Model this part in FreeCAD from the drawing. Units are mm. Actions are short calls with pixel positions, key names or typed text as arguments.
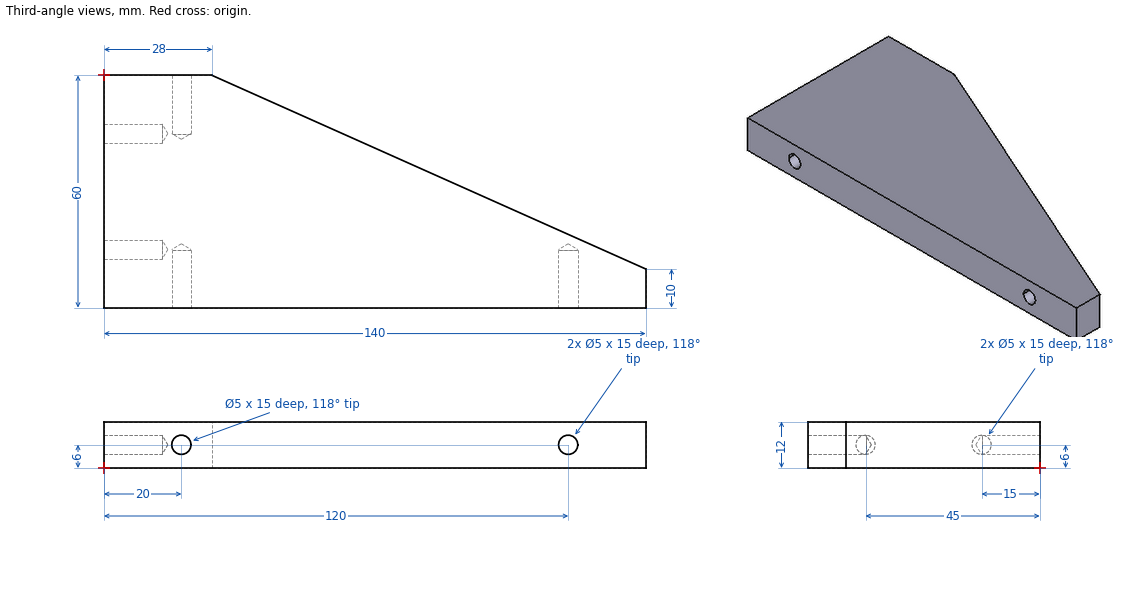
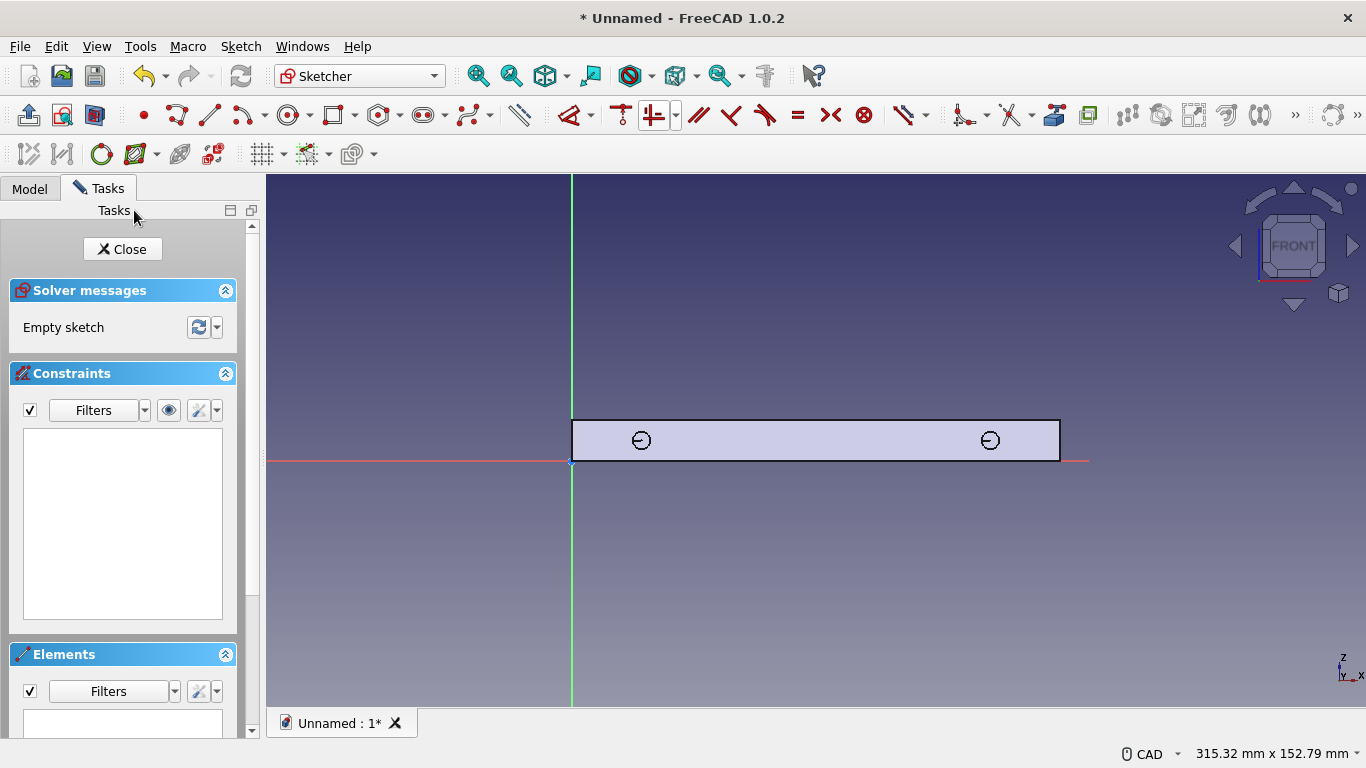
key(q)
key(s)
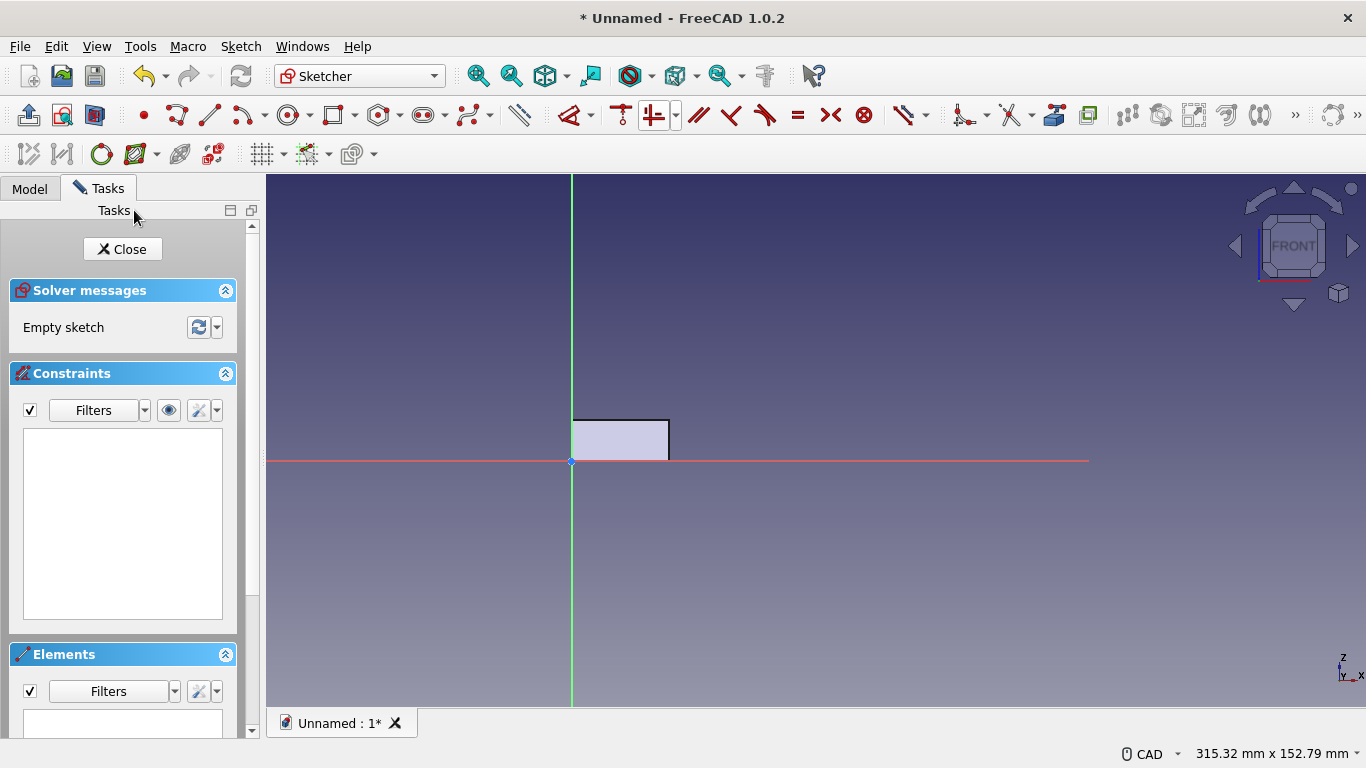
scroll(636, 440, up, 15)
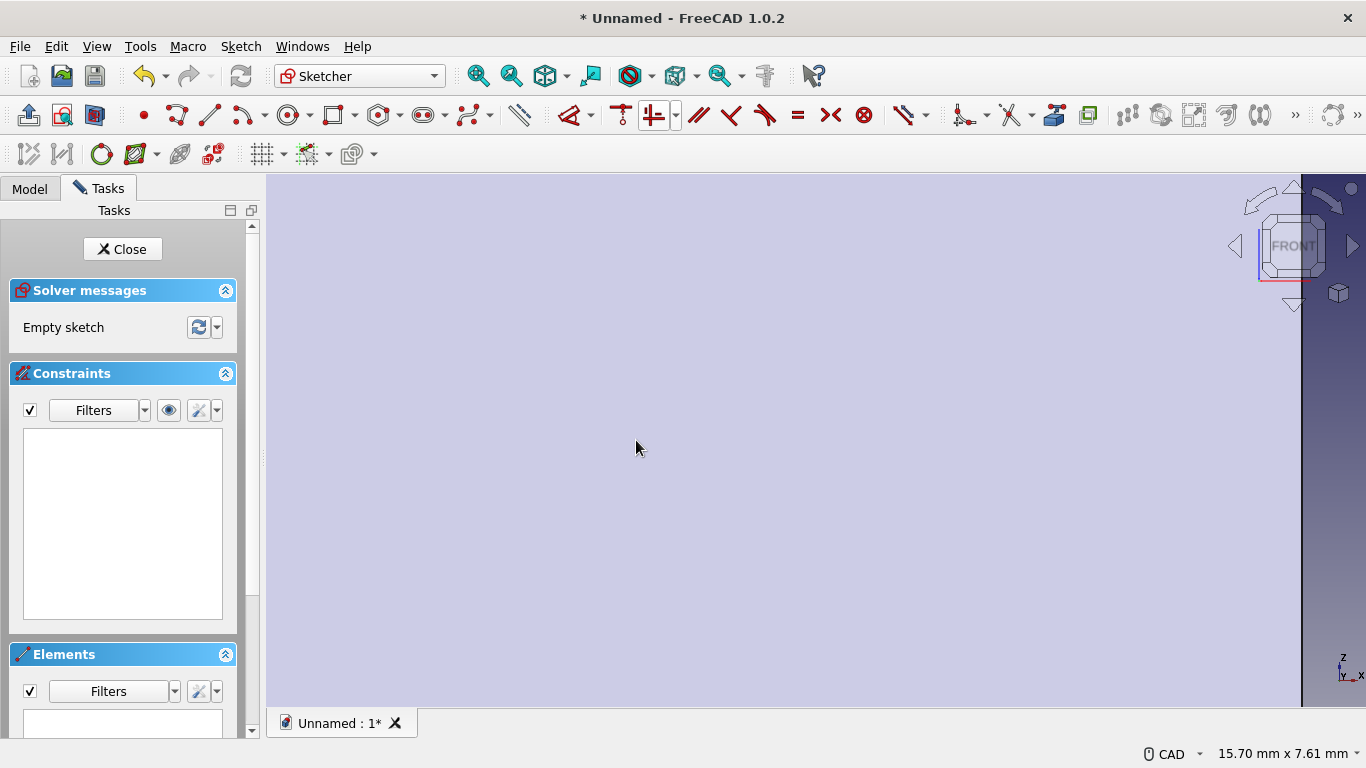
click(288, 116)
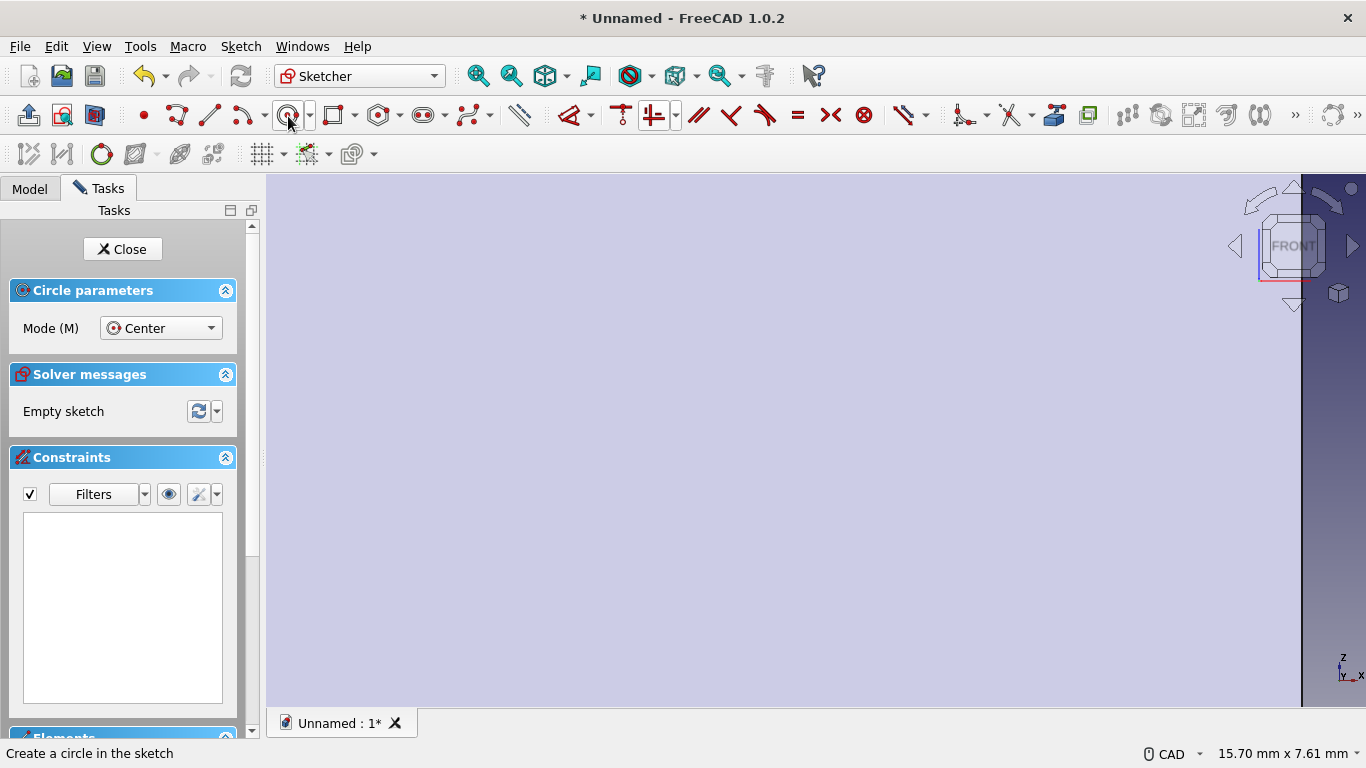
click(742, 440)
move(865, 317)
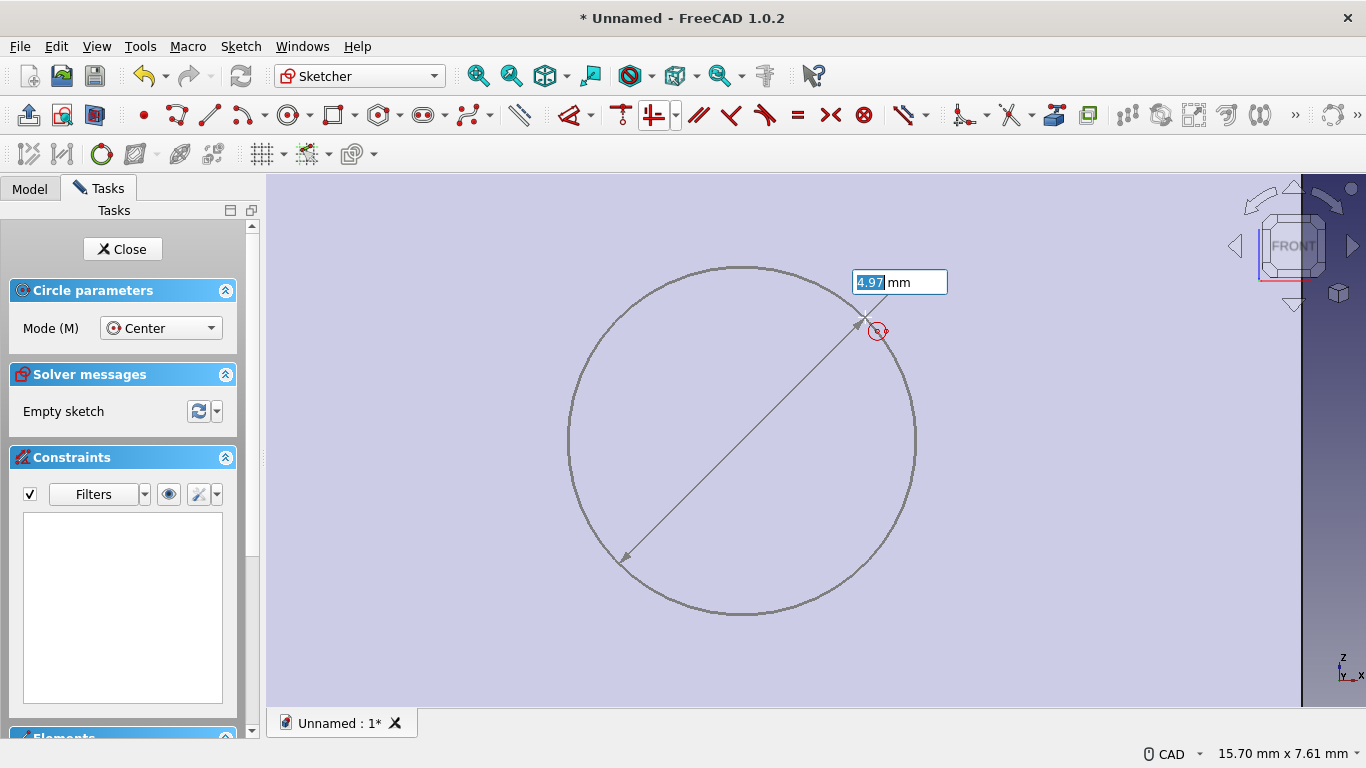
text(5)
key(Return)
key(Escape)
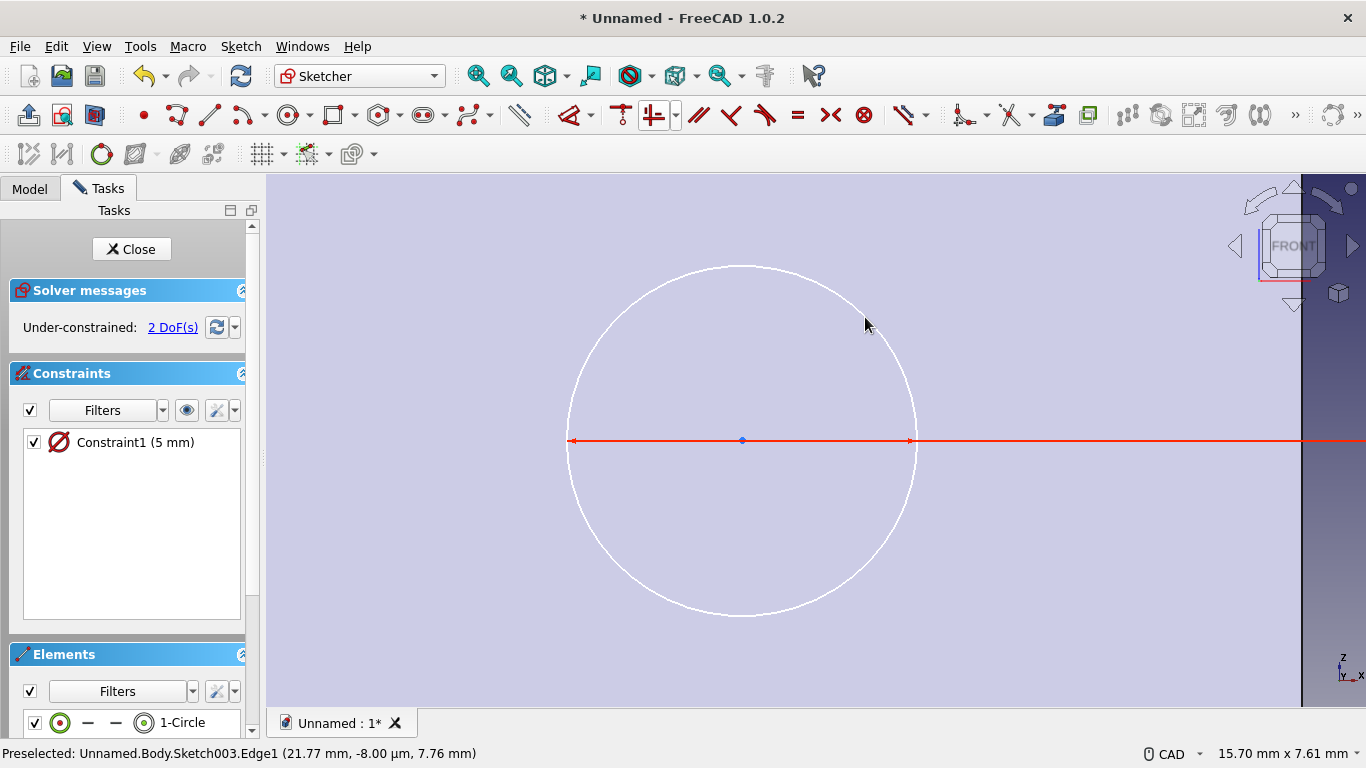
key(d)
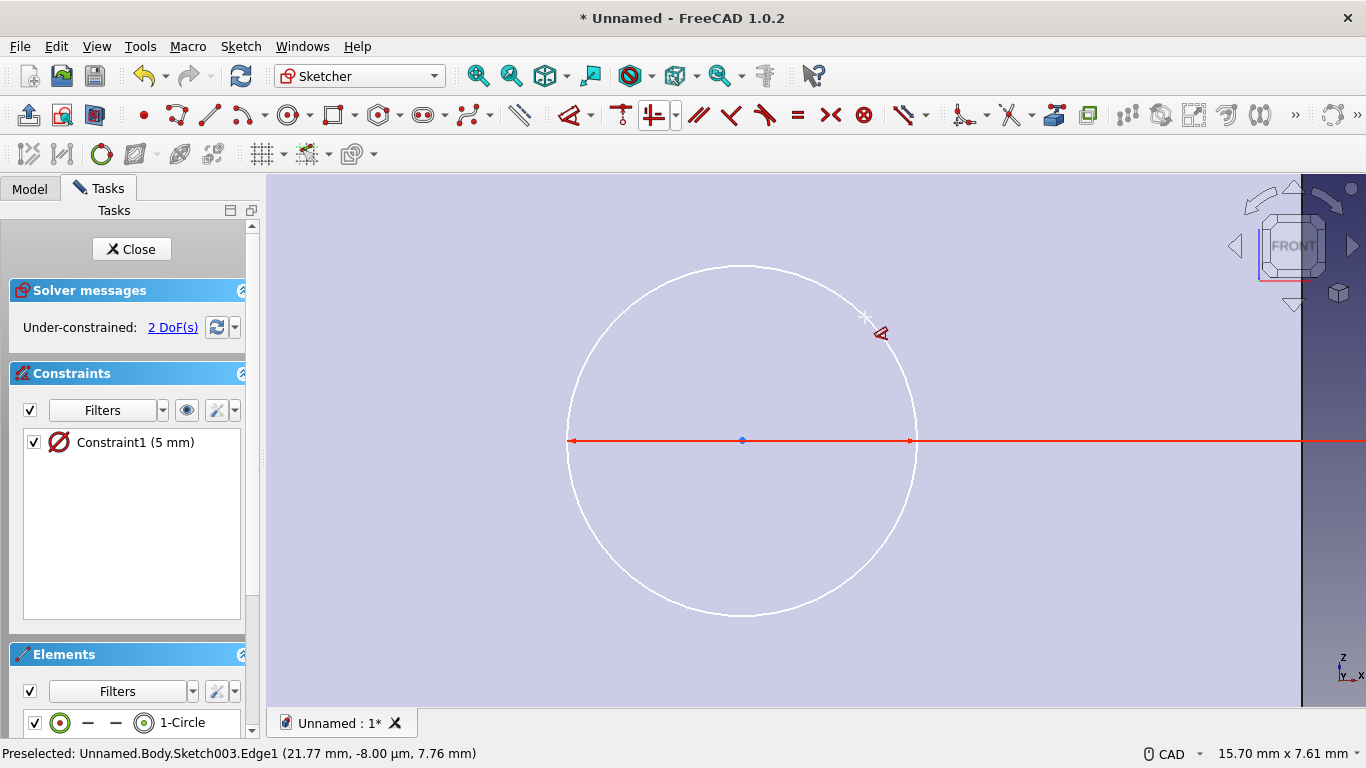
click(742, 441)
click(776, 560)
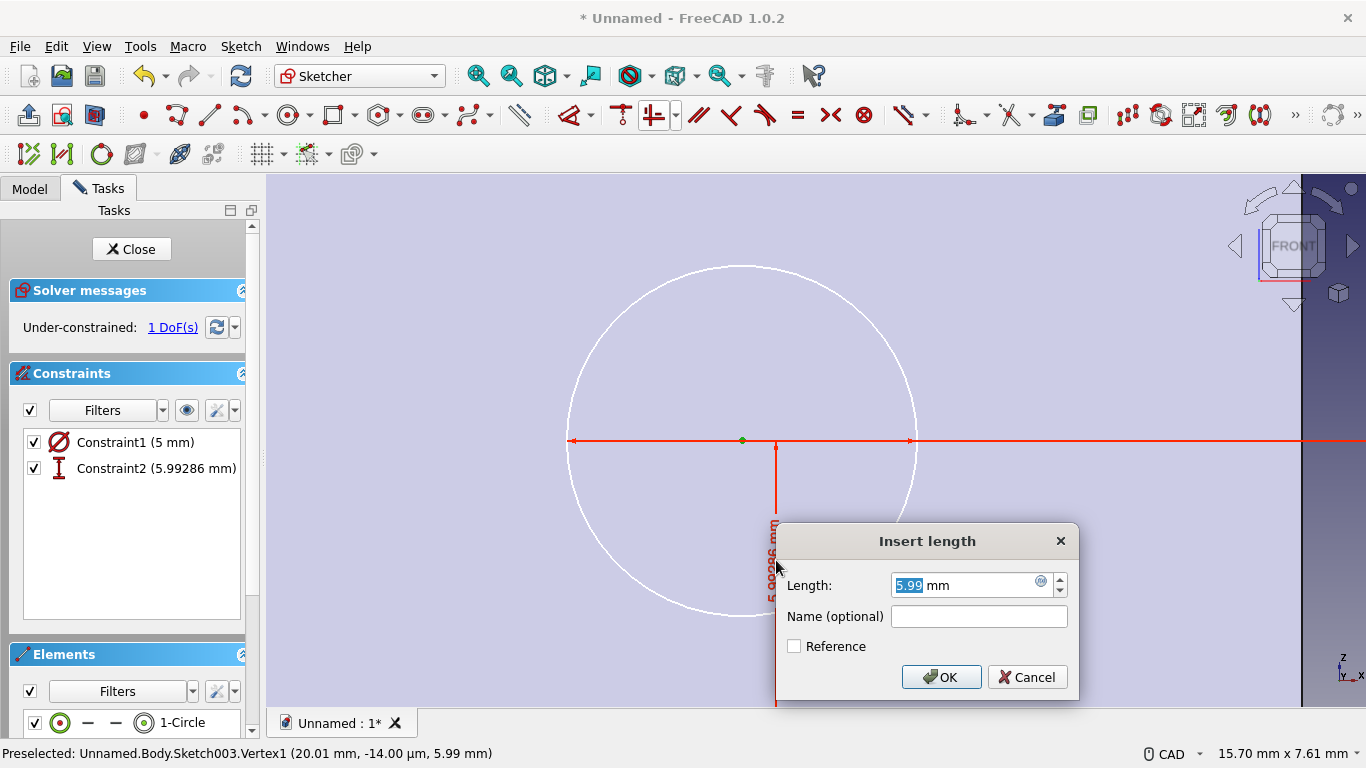
text(6)
key(Return)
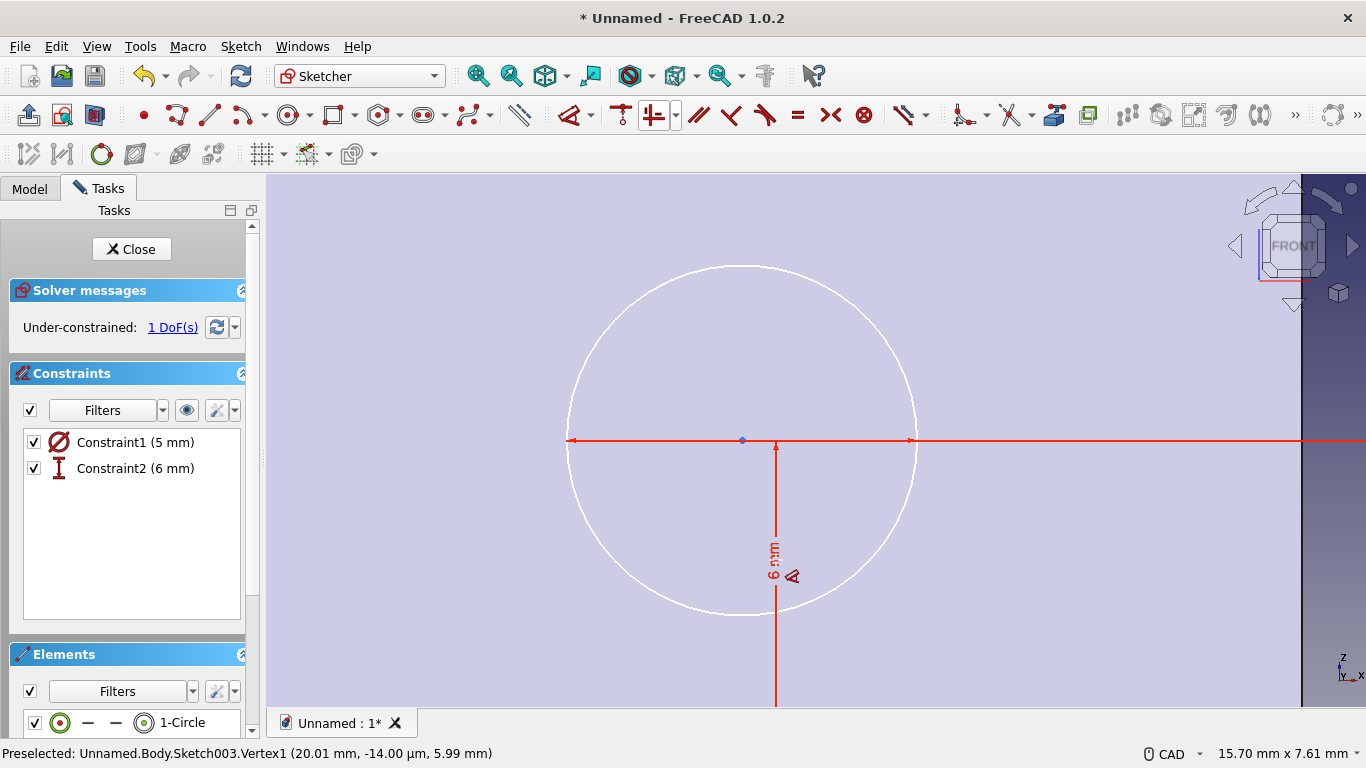
click(742, 440)
click(518, 406)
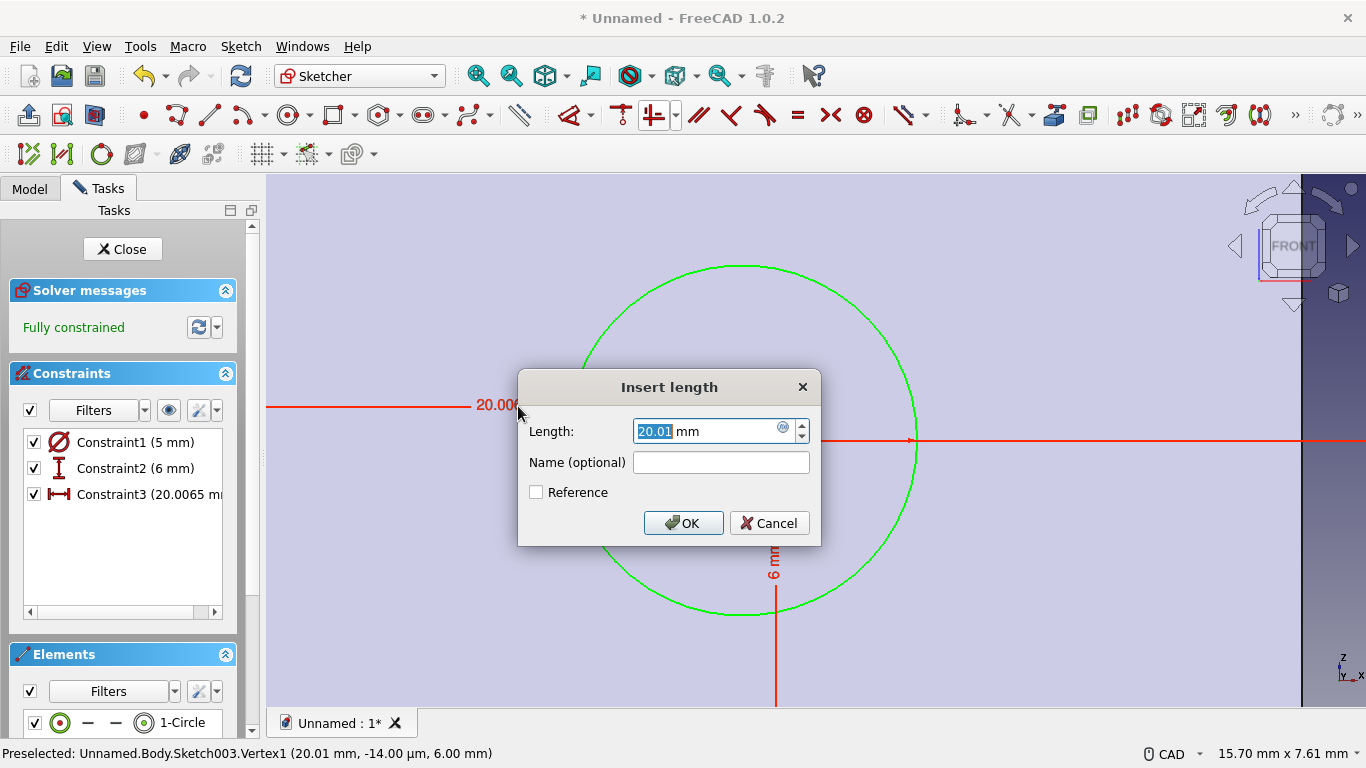
text(20)
key(Return)
key(Escape)